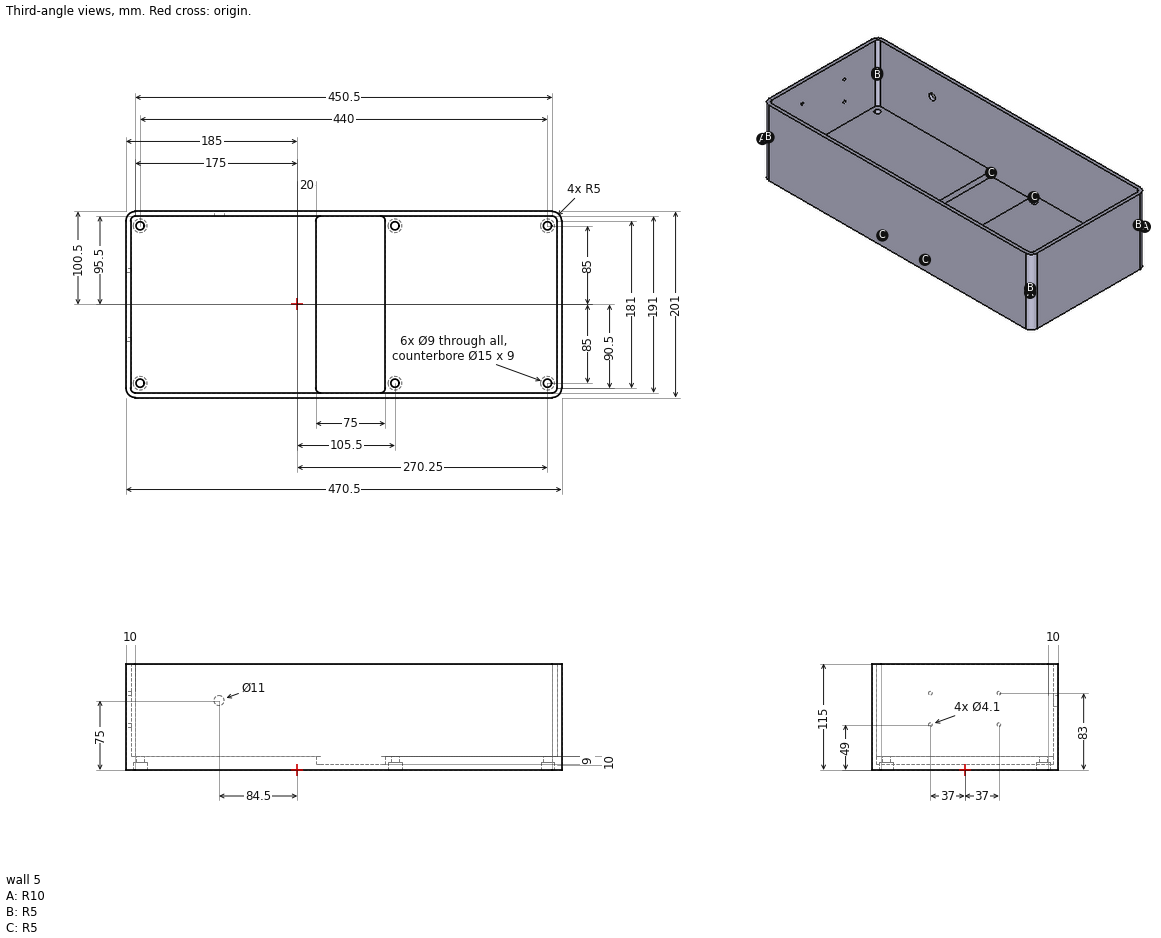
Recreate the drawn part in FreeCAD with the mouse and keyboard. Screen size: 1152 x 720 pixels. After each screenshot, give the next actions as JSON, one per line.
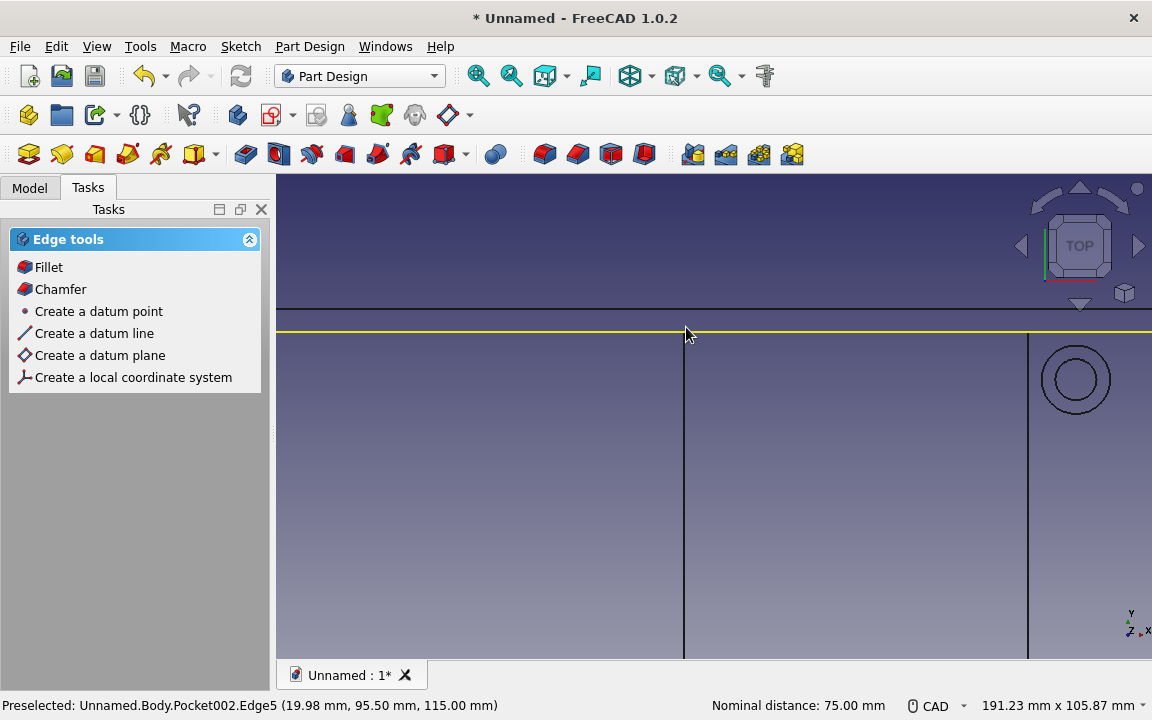
{"action": "key", "text": "v f"}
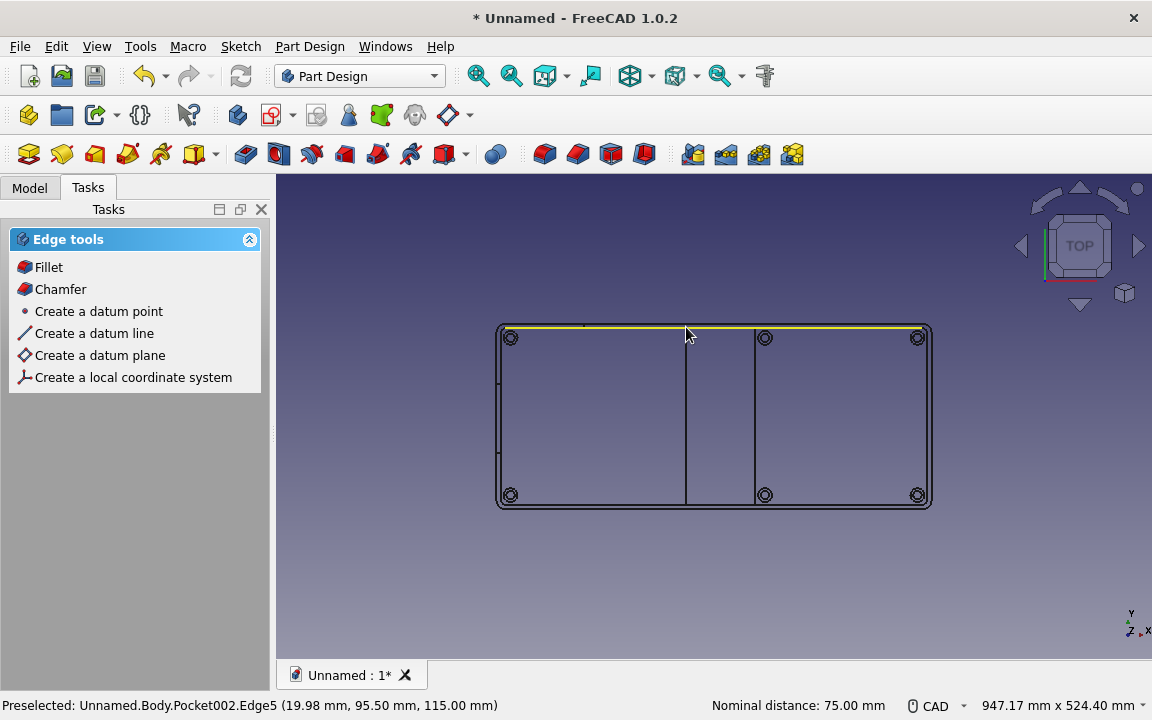
{"action": "key", "text": "1"}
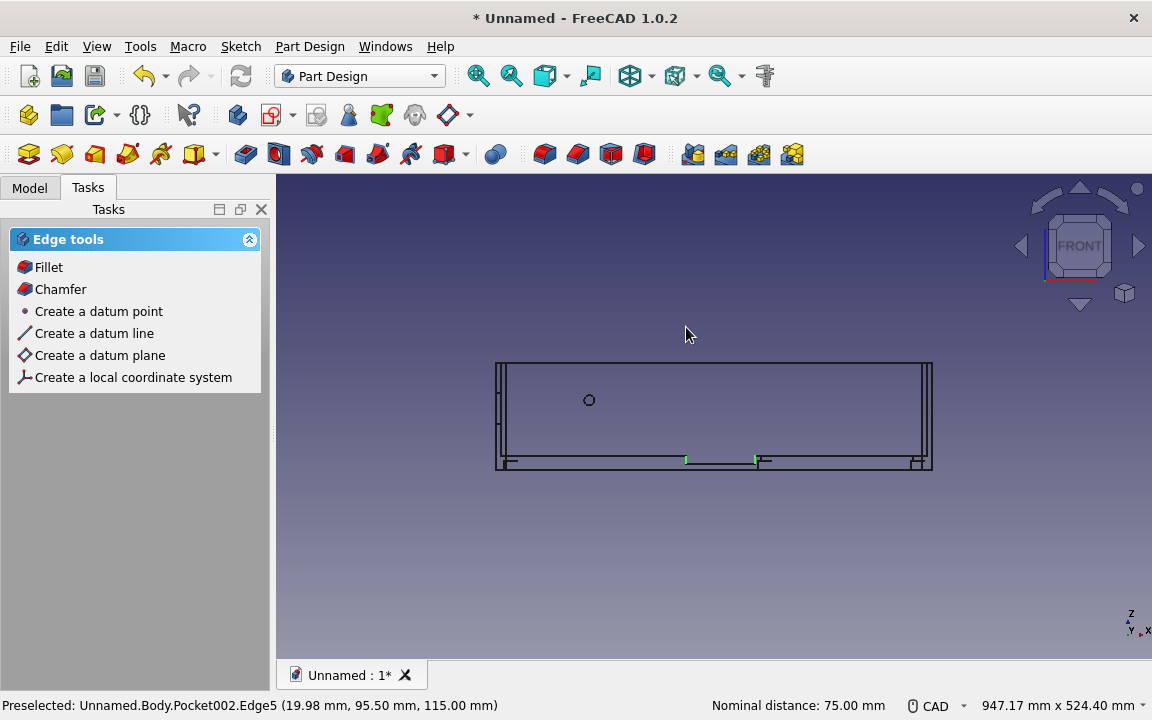
{"action": "scroll", "coordinate": [686, 459], "scroll_direction": "up", "scroll_amount": 8}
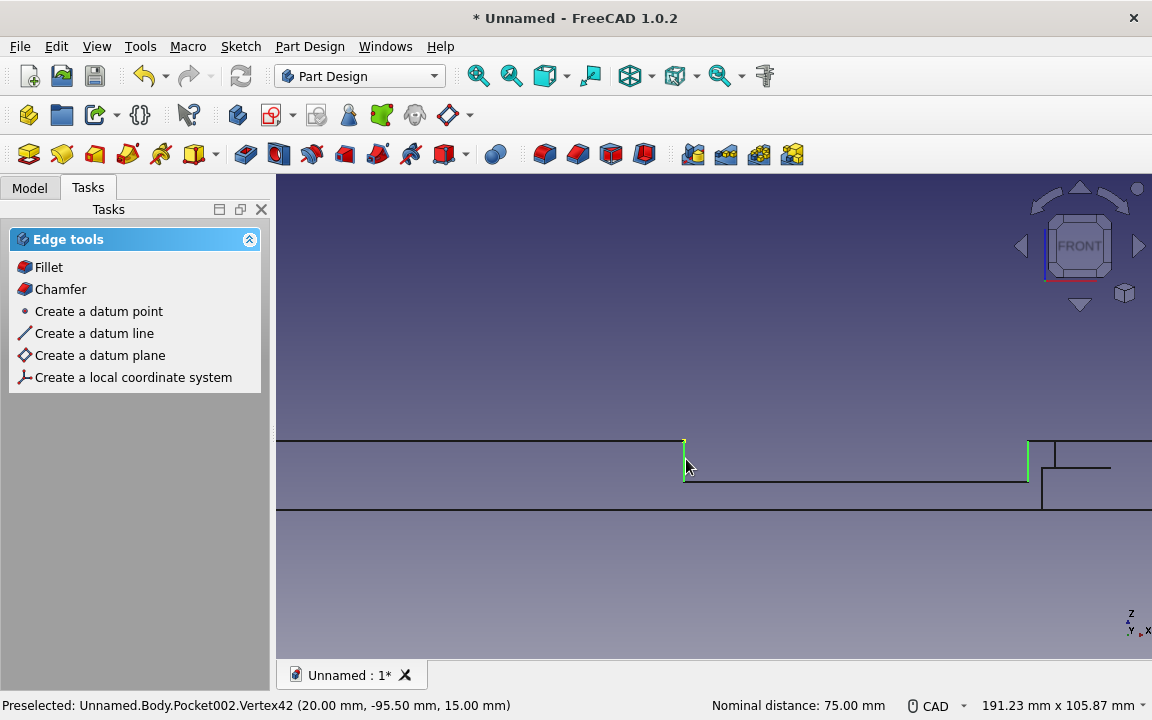
{"action": "key", "text": "v f"}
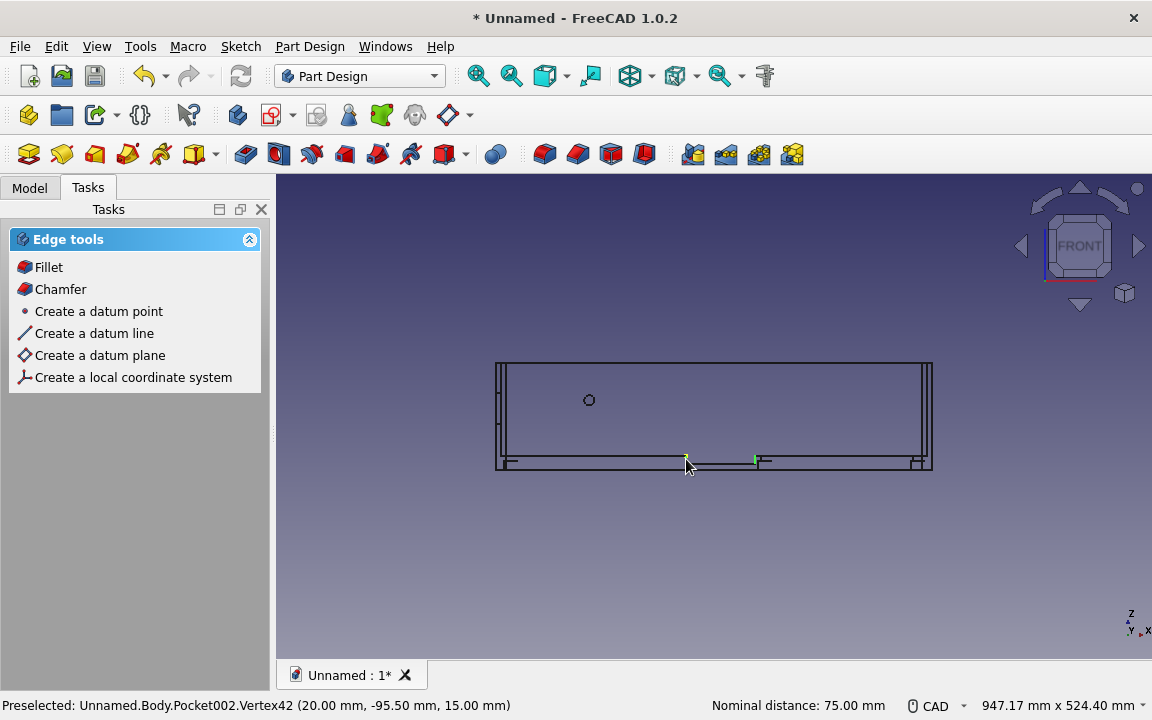
{"action": "key", "text": "3"}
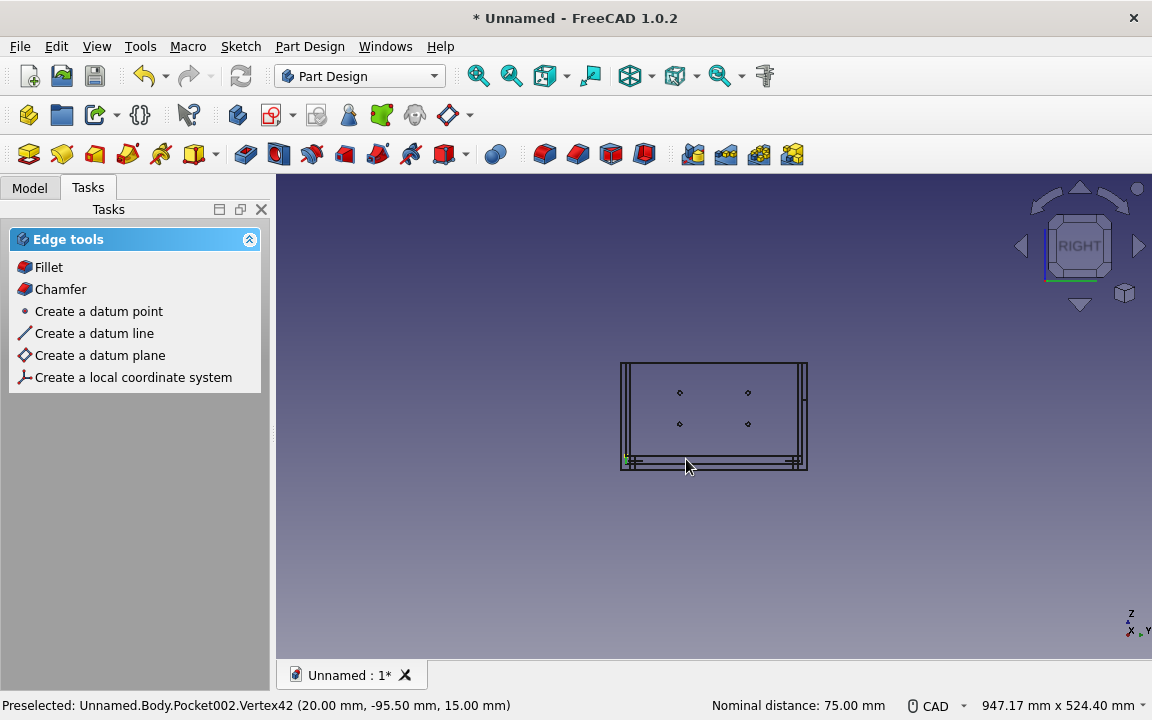
{"action": "key", "text": "v f"}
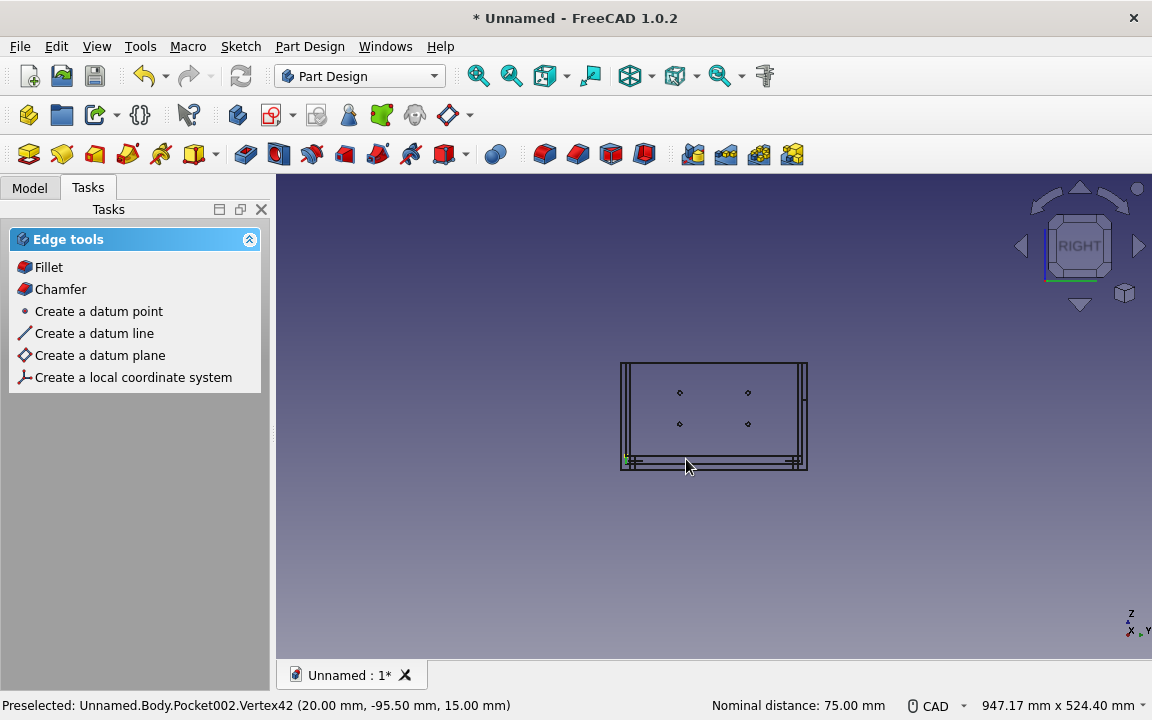
{"action": "scroll", "coordinate": [802, 459], "scroll_direction": "up", "scroll_amount": 8}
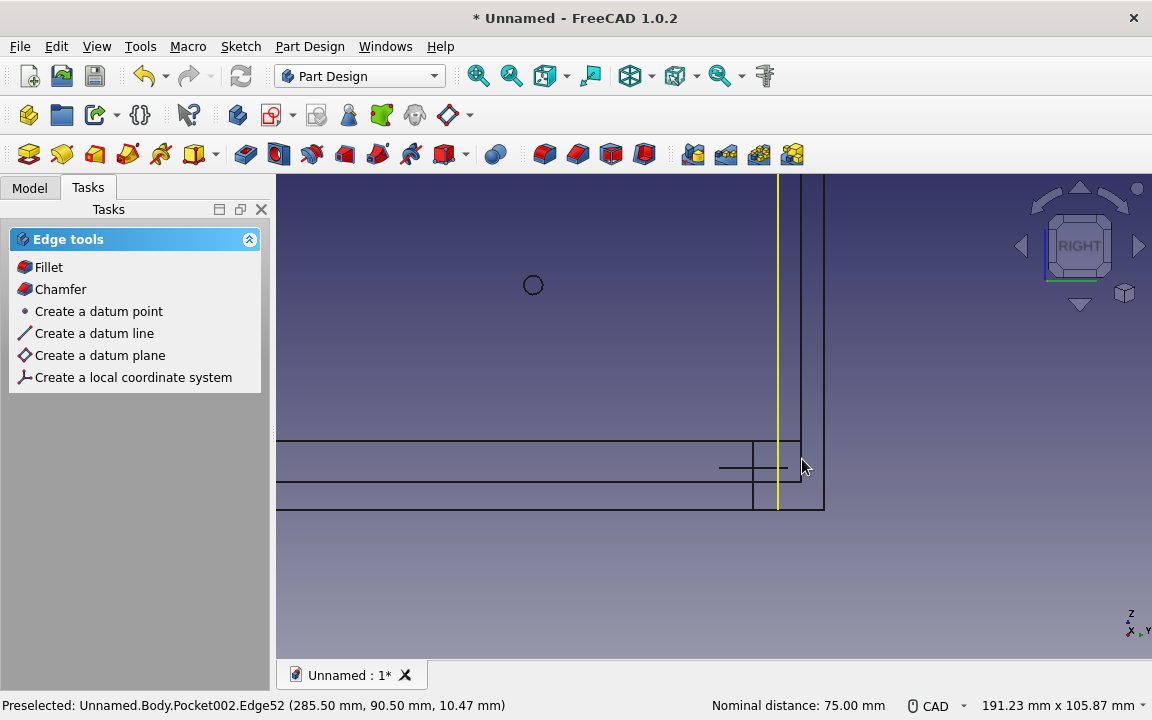
{"action": "left_click", "coordinate": [801, 460], "text": "ctrl"}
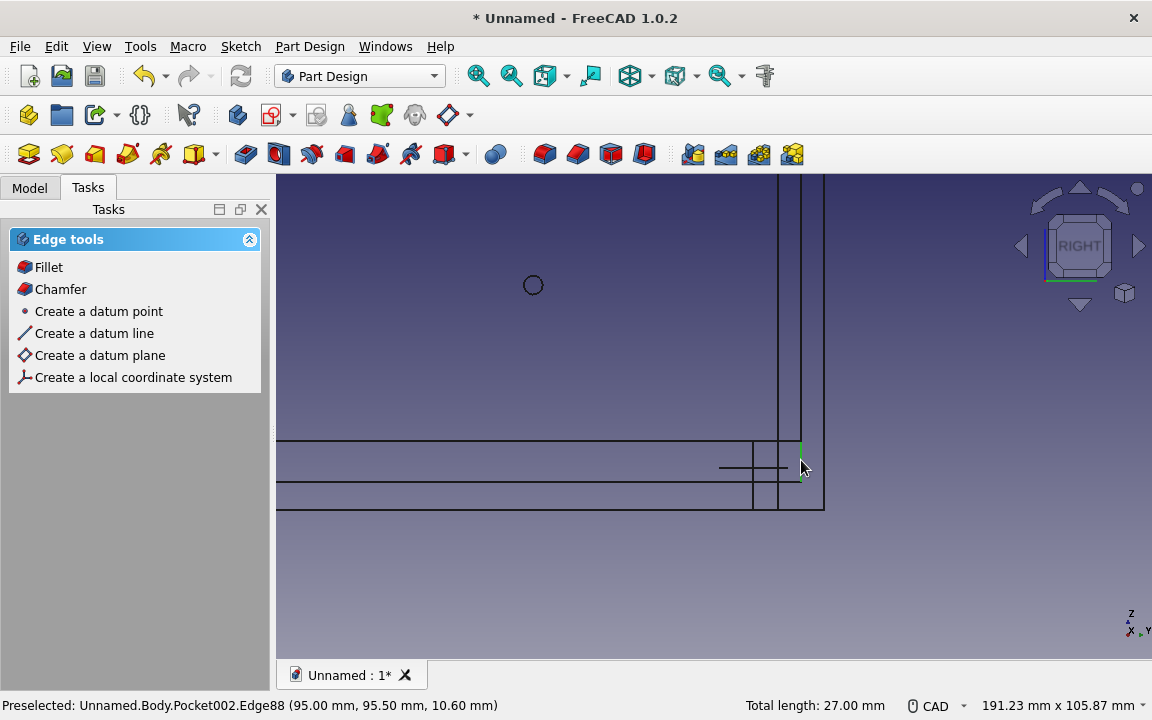
{"action": "key", "text": "v f"}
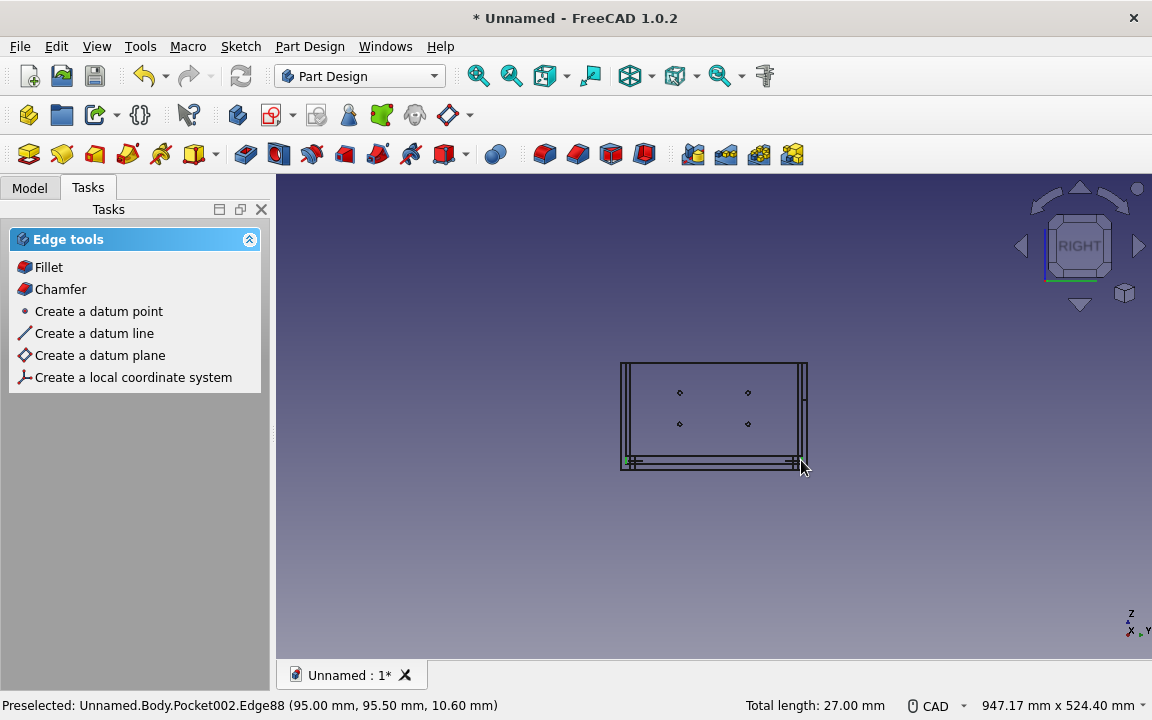
{"action": "key", "text": "5"}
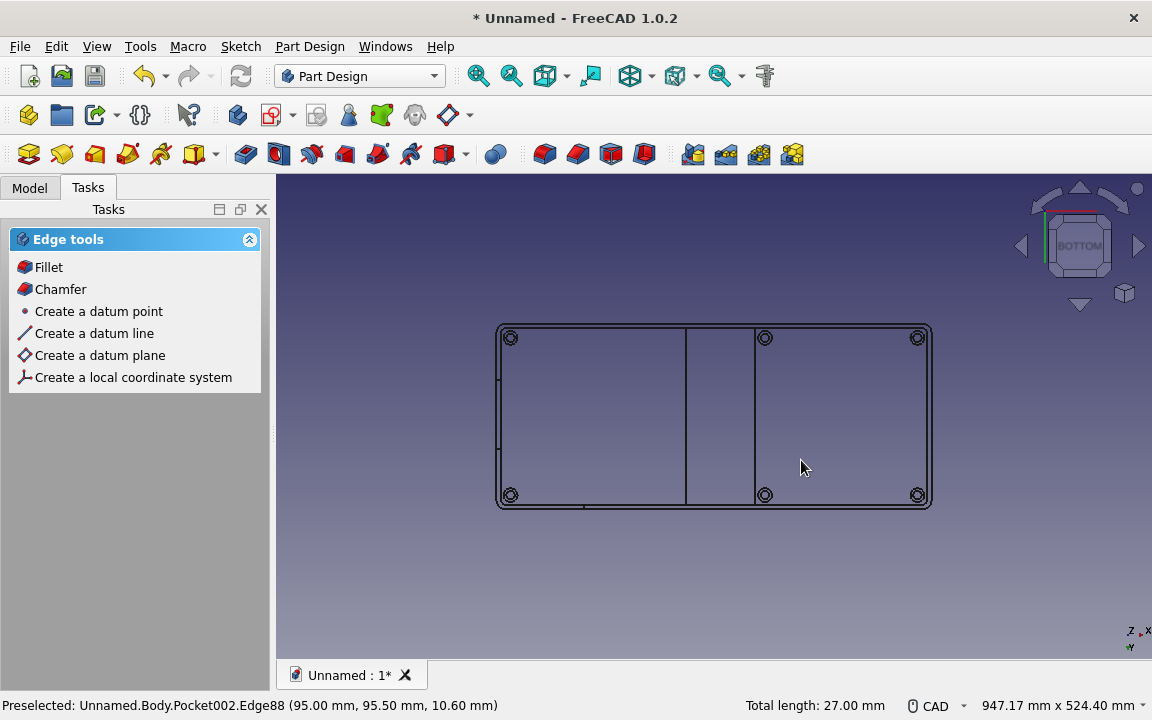
{"action": "scroll", "coordinate": [686, 504], "scroll_direction": "up", "scroll_amount": 8}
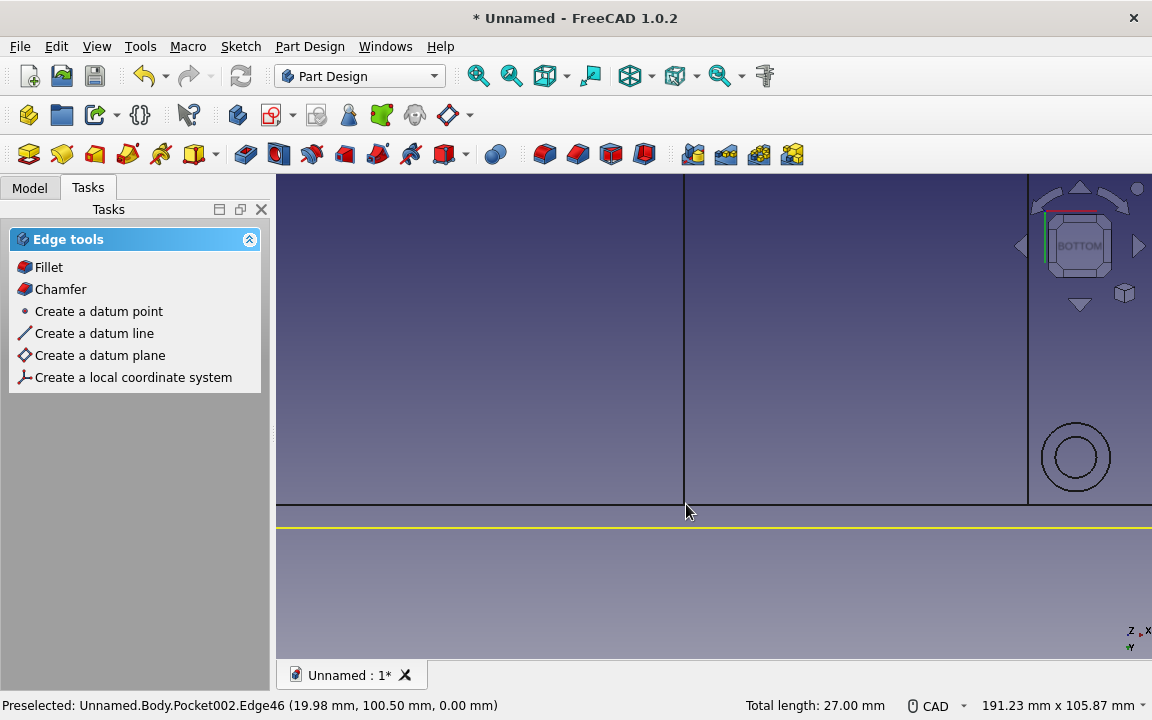
{"action": "key", "text": "v f"}